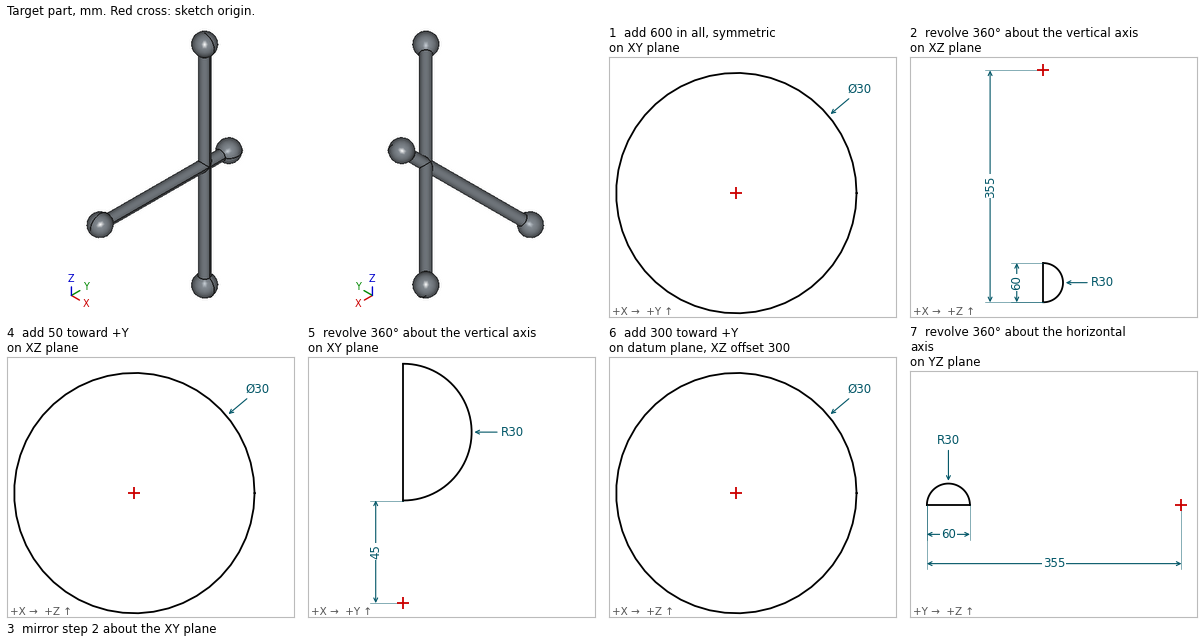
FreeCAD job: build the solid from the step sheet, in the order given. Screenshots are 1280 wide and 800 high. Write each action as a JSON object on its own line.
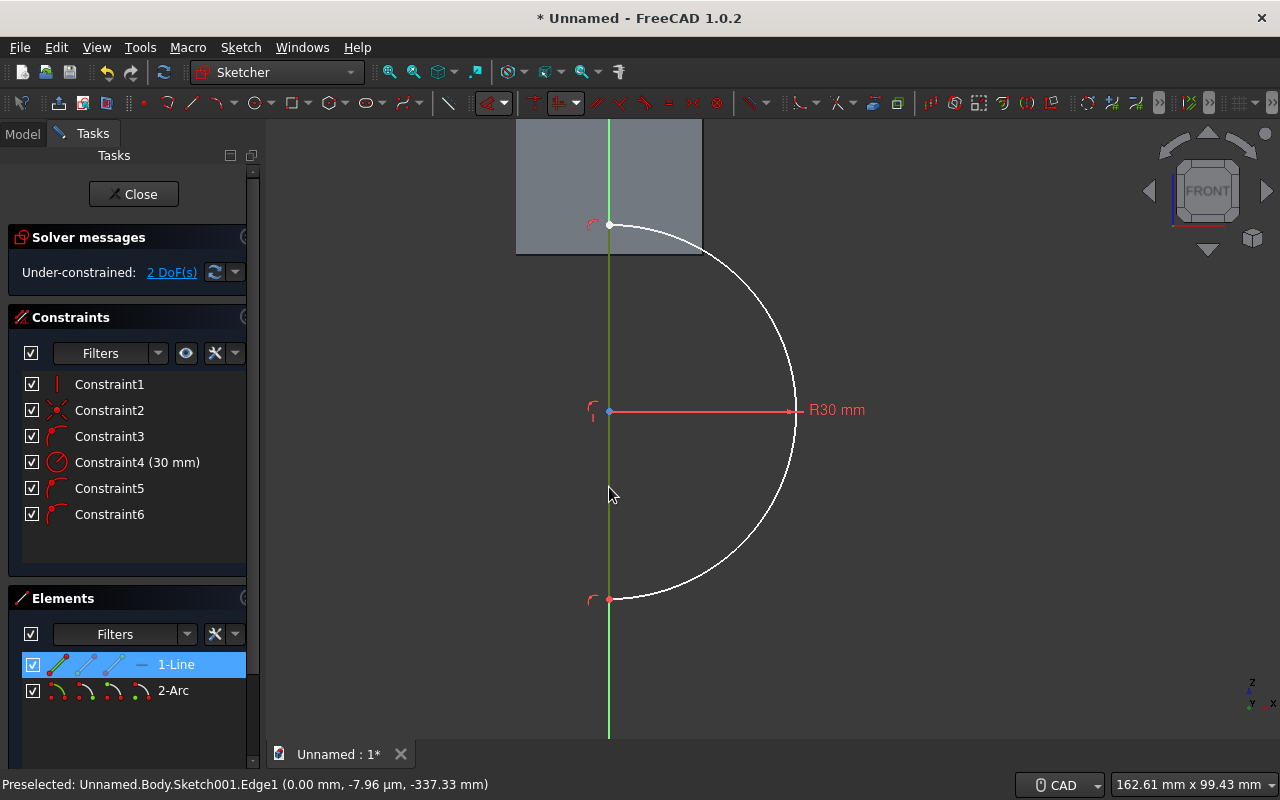
{"action": "key", "text": "i"}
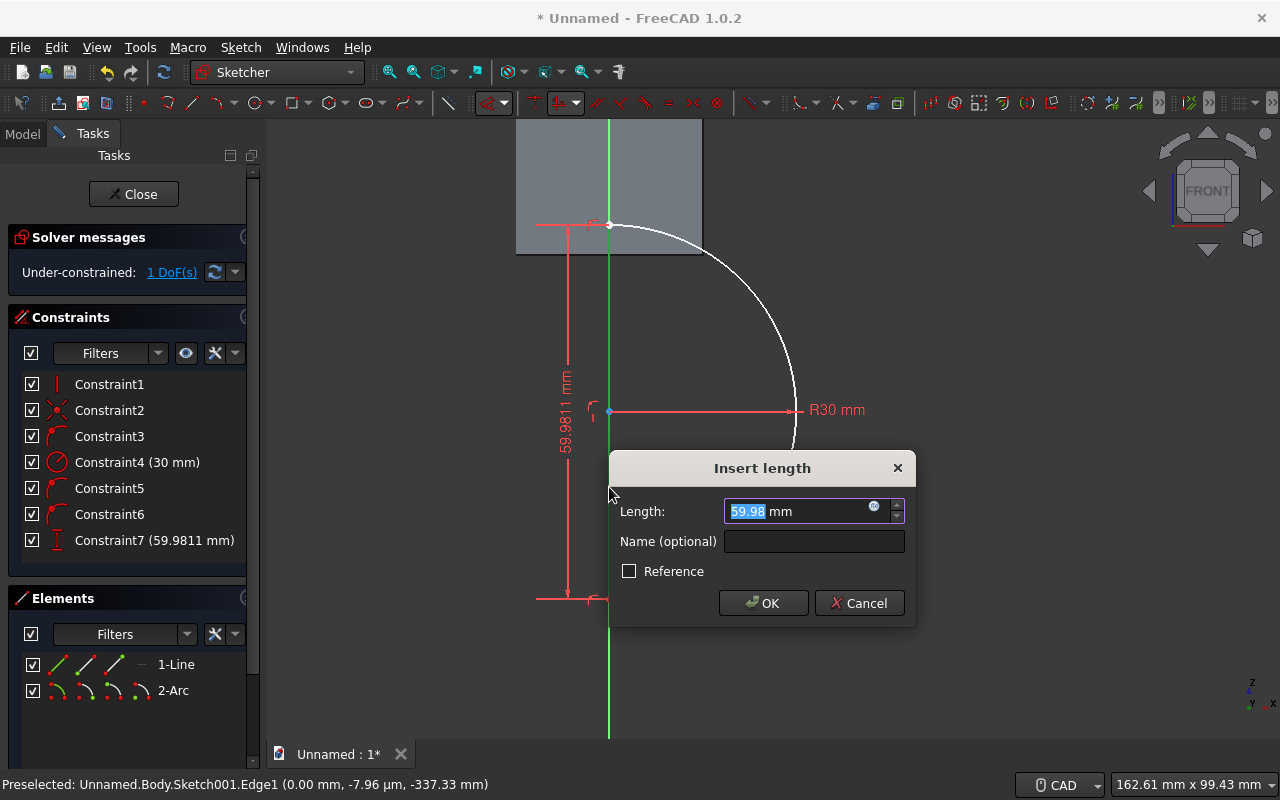
{"action": "type", "text": "60"}
{"action": "key", "text": "Return"}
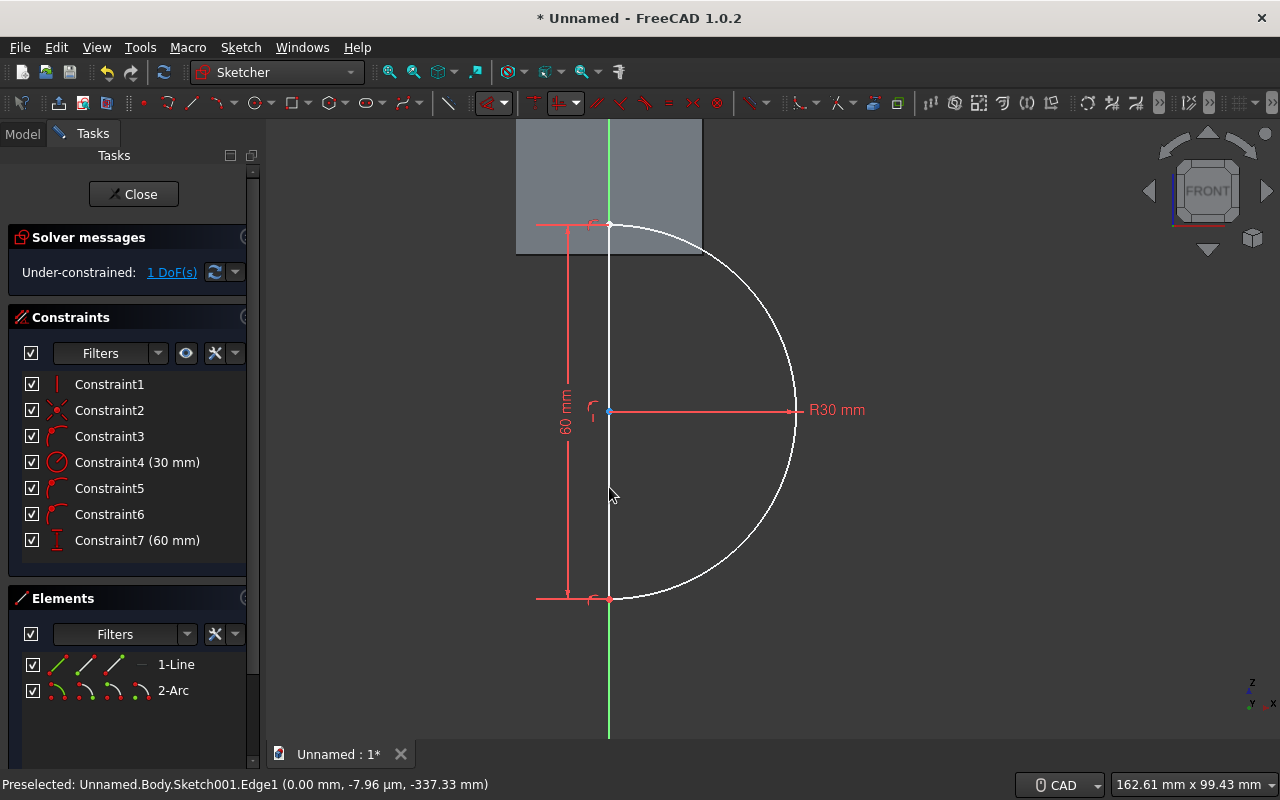
{"action": "left_click", "coordinate": [609, 599]}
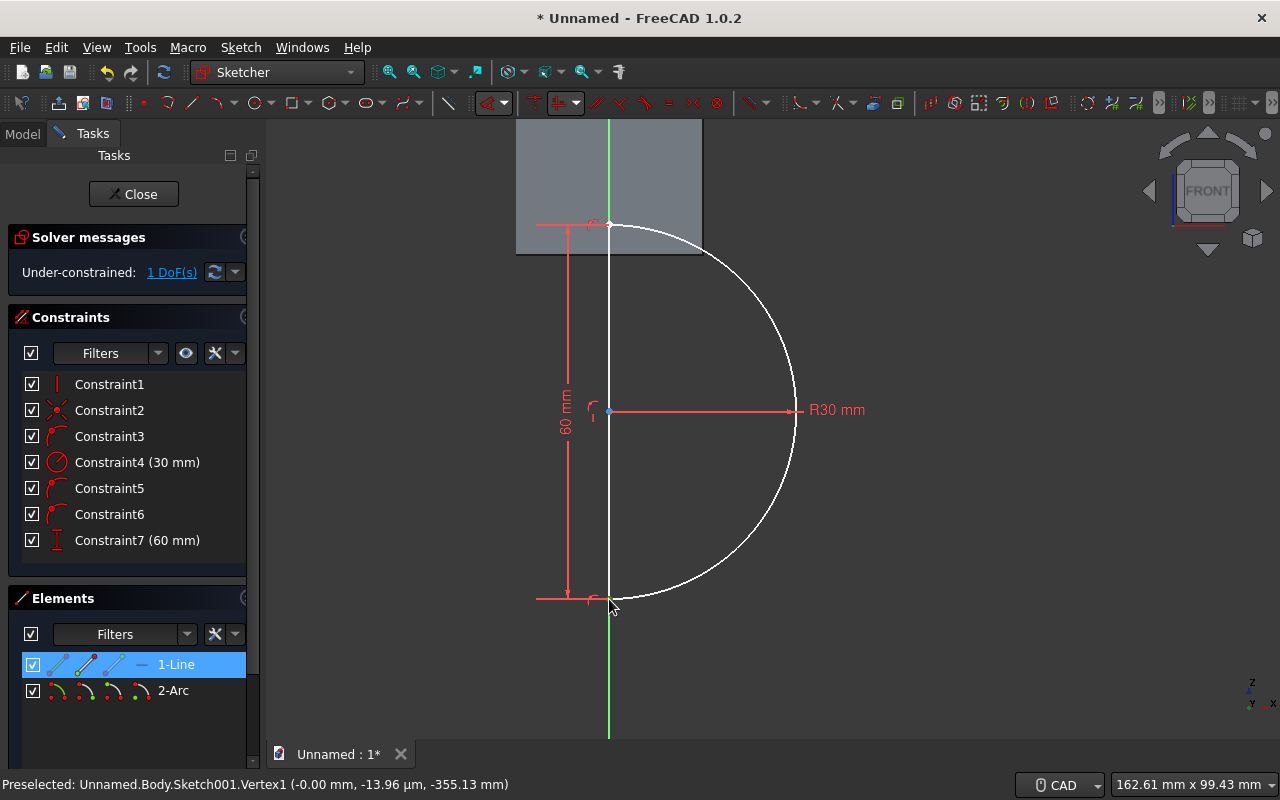
{"action": "key", "text": "i"}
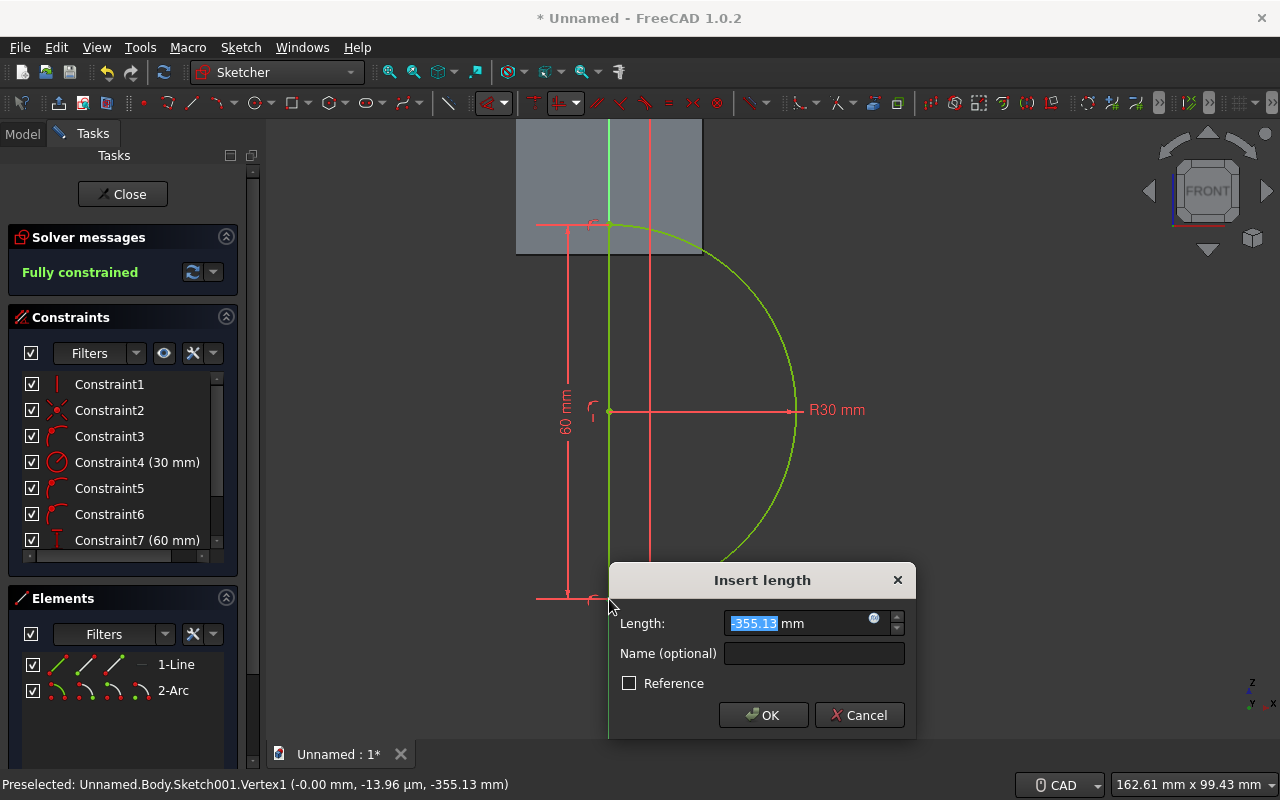
{"action": "type", "text": "-355"}
{"action": "key", "text": "Return"}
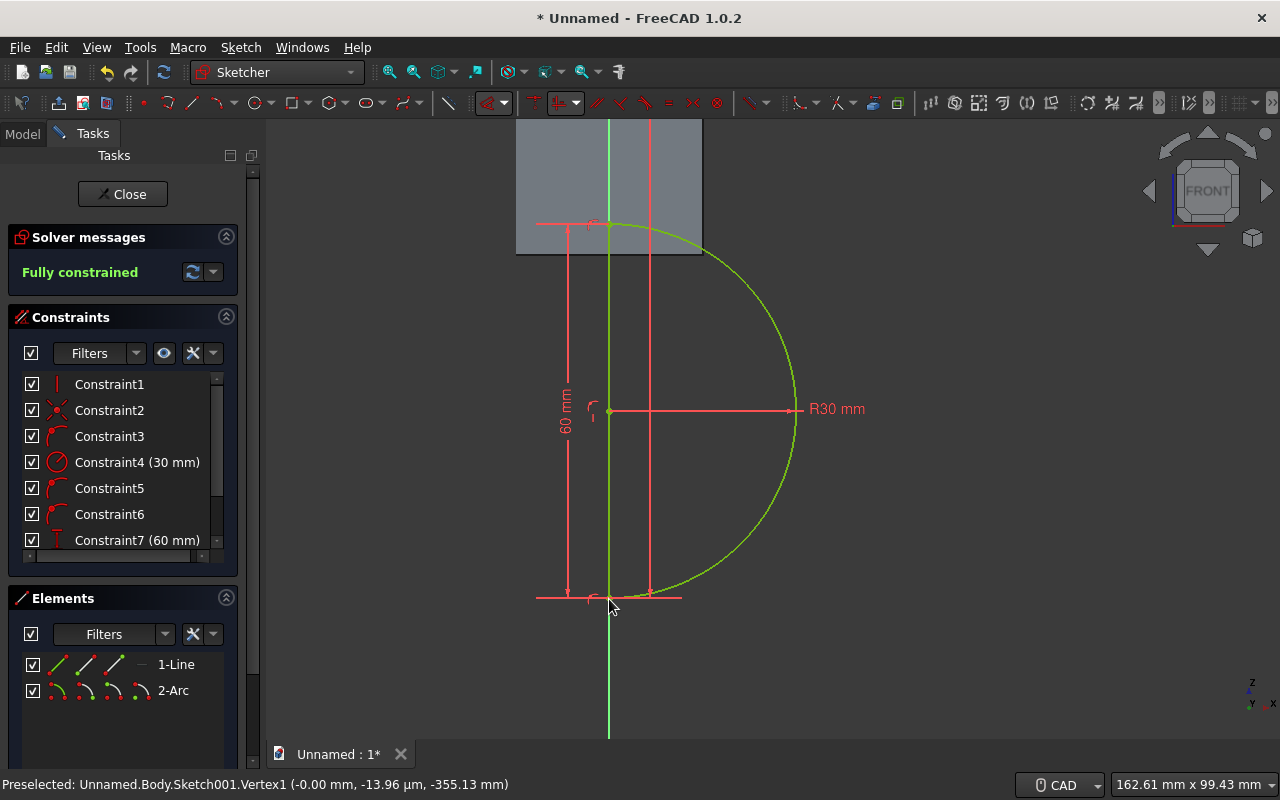
{"action": "left_click", "coordinate": [123, 194]}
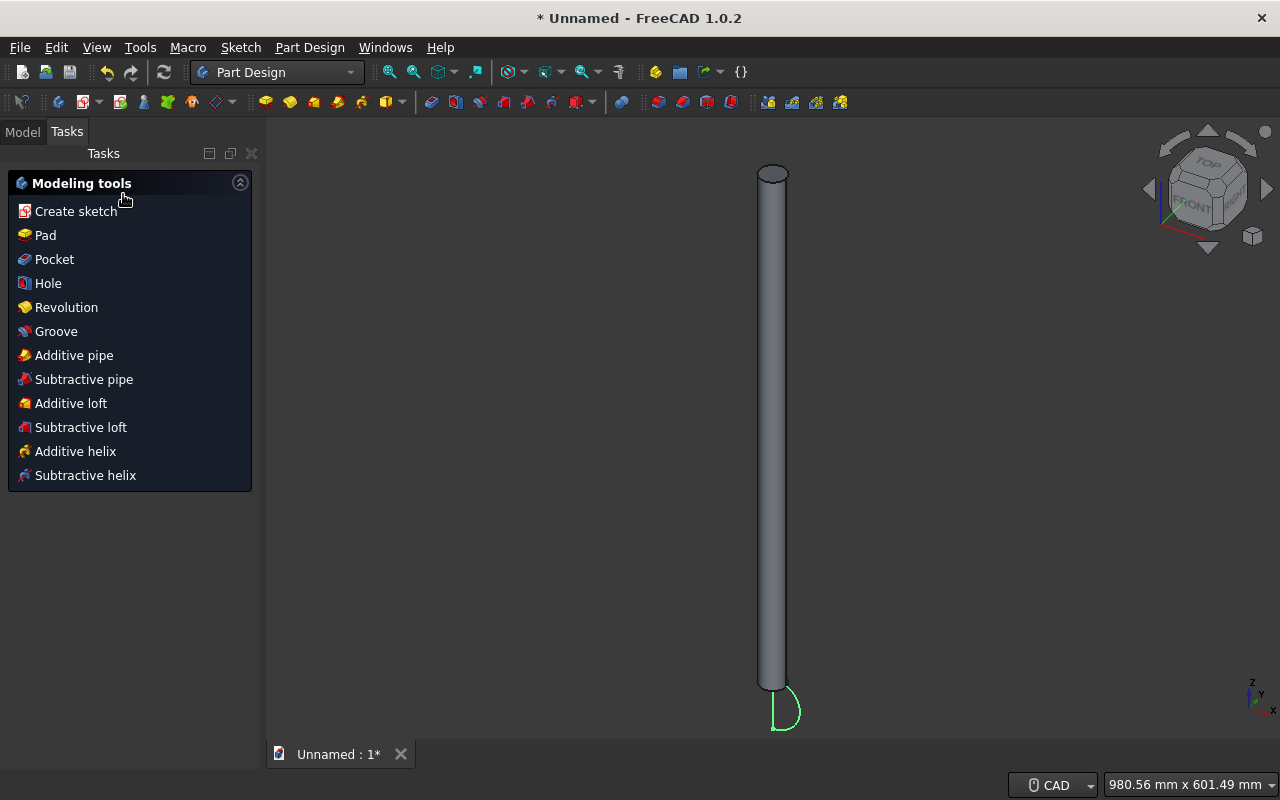
{"action": "left_click", "coordinate": [290, 102]}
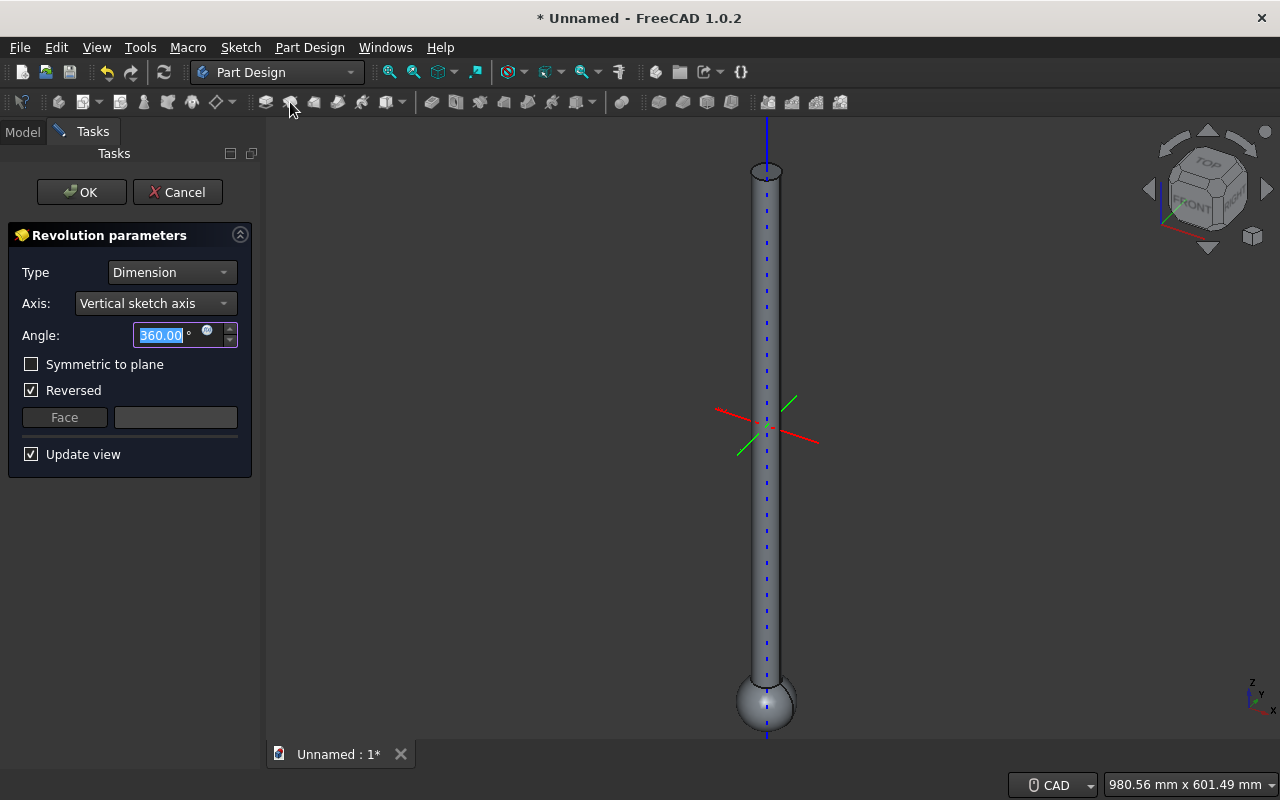
{"action": "left_click", "coordinate": [82, 192]}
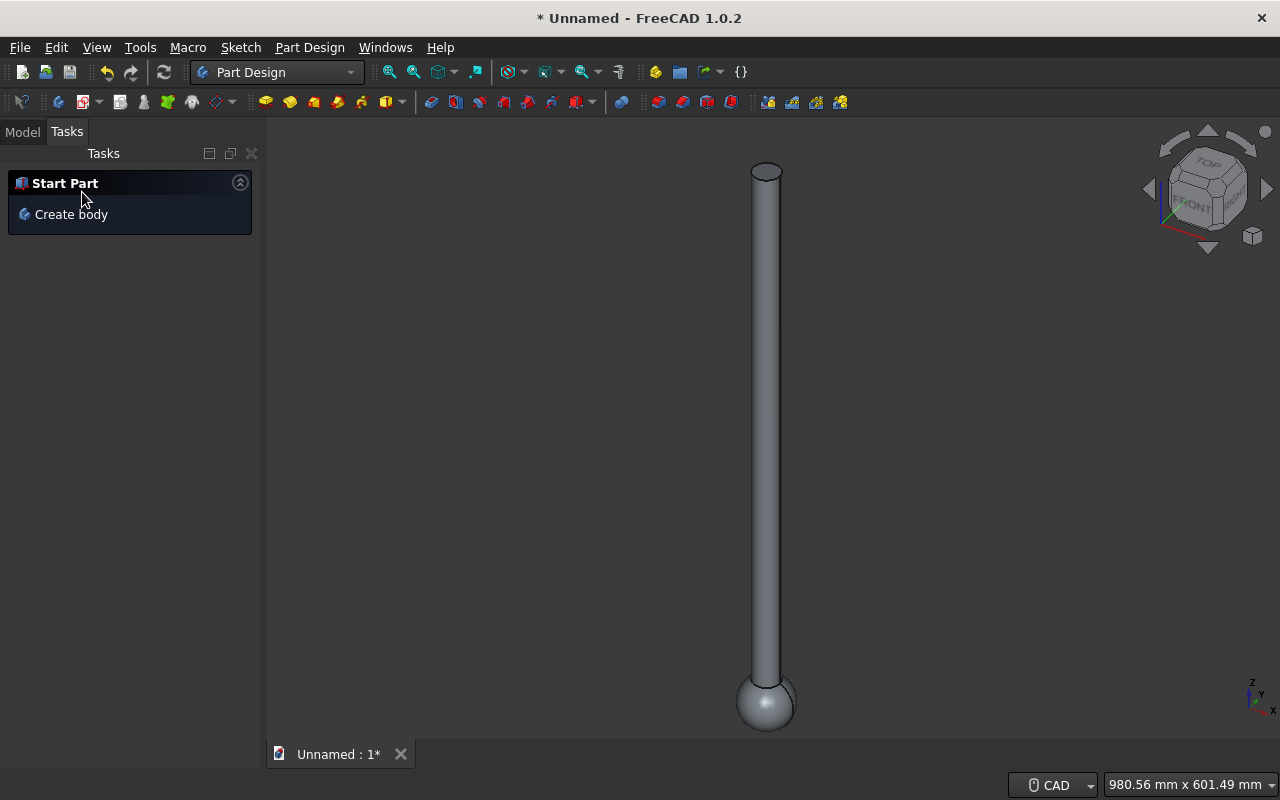
{"action": "left_click", "coordinate": [390, 72]}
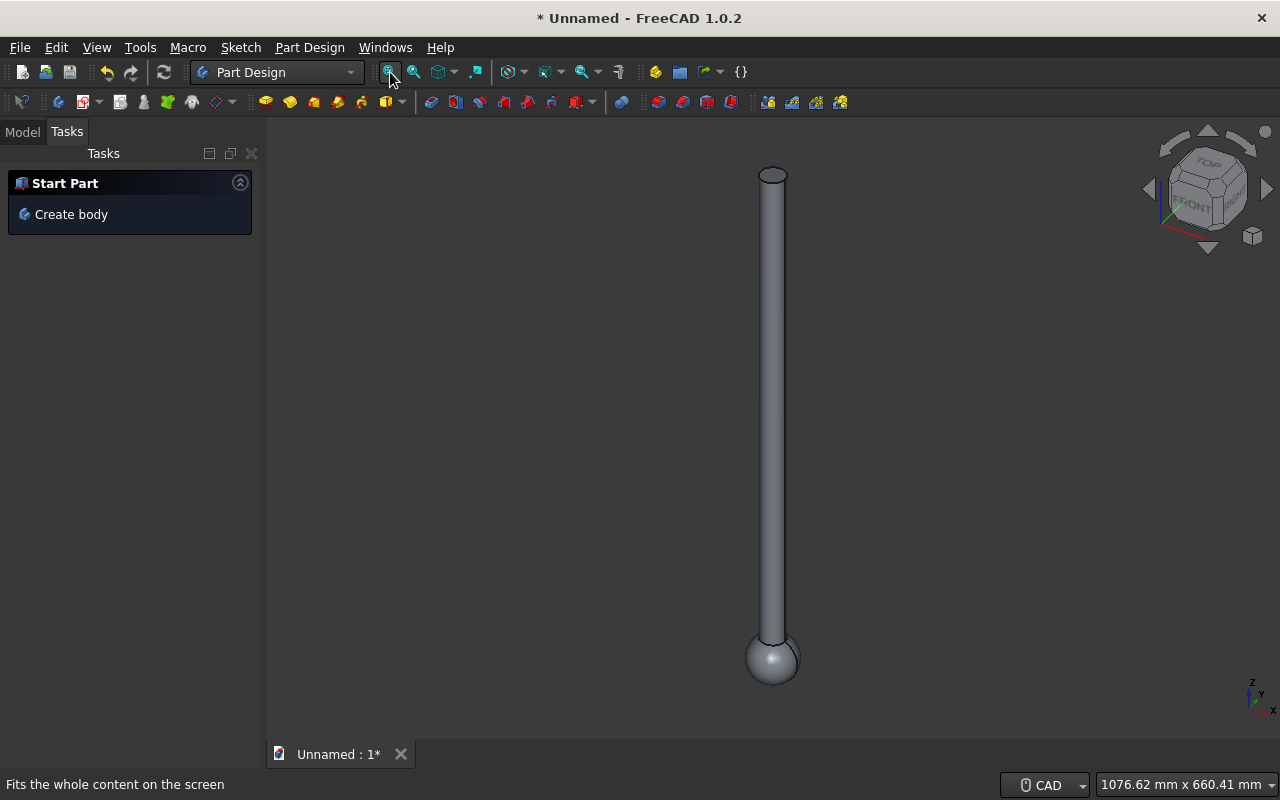
{"action": "left_click", "coordinate": [23, 131]}